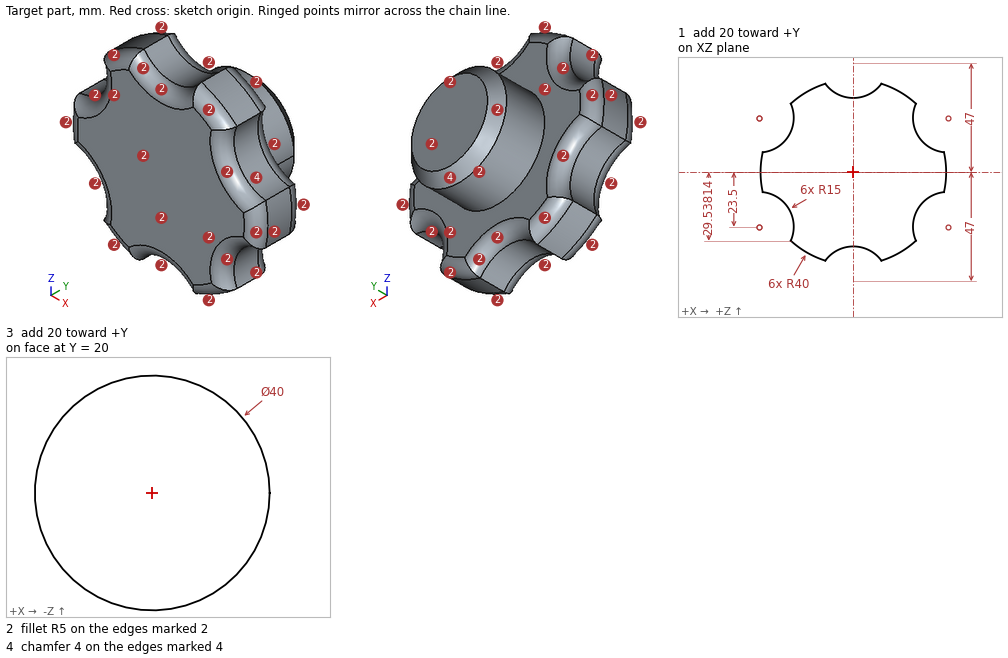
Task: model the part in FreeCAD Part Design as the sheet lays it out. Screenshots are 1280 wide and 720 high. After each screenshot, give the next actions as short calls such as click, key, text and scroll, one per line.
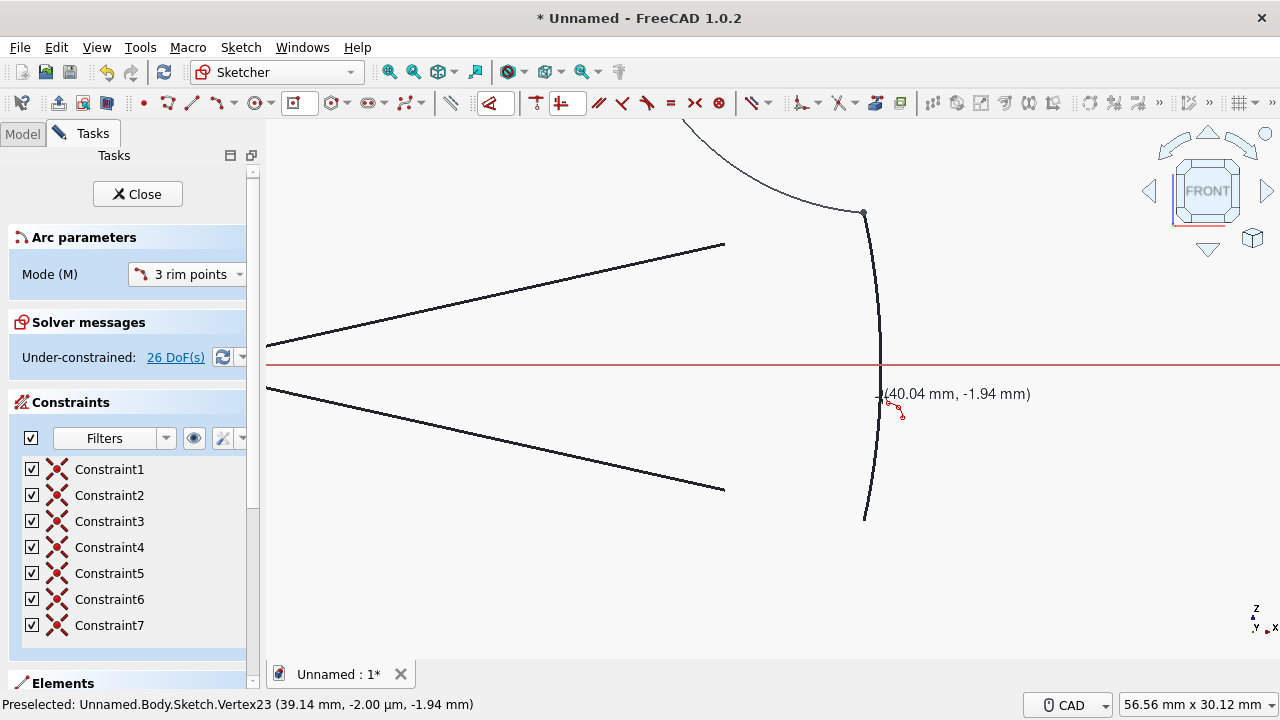
click(879, 396)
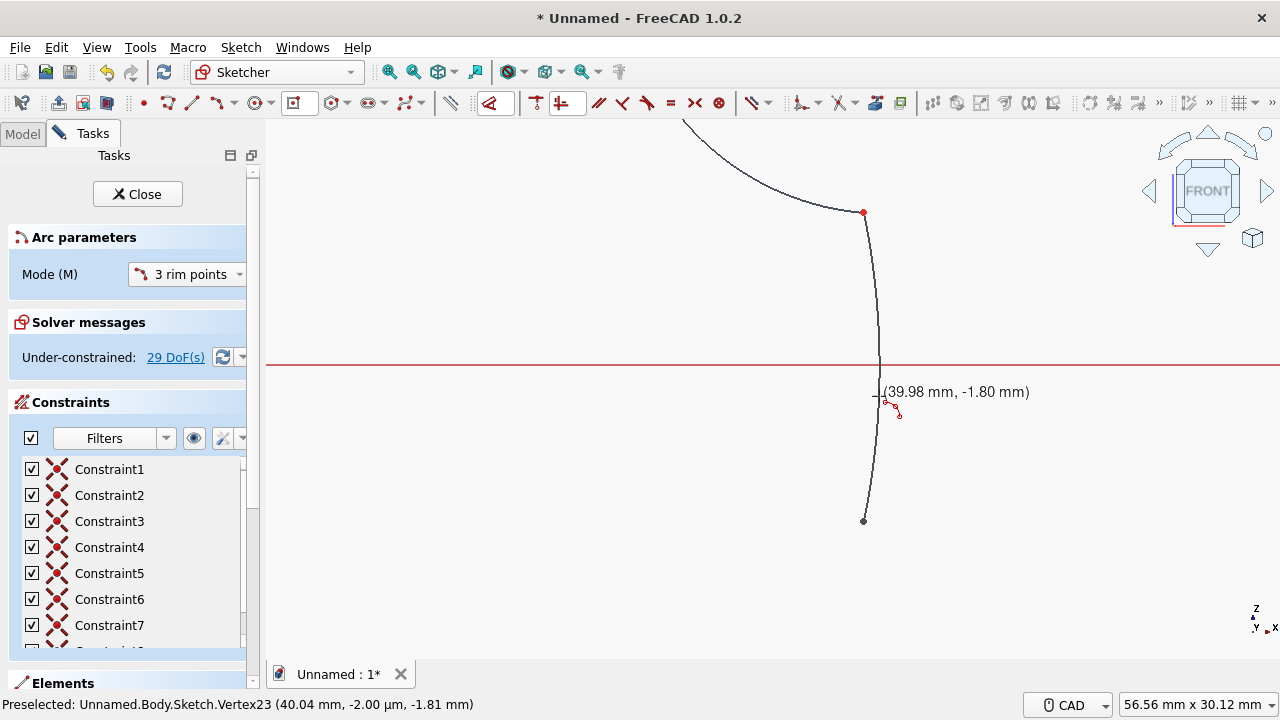
click(864, 521)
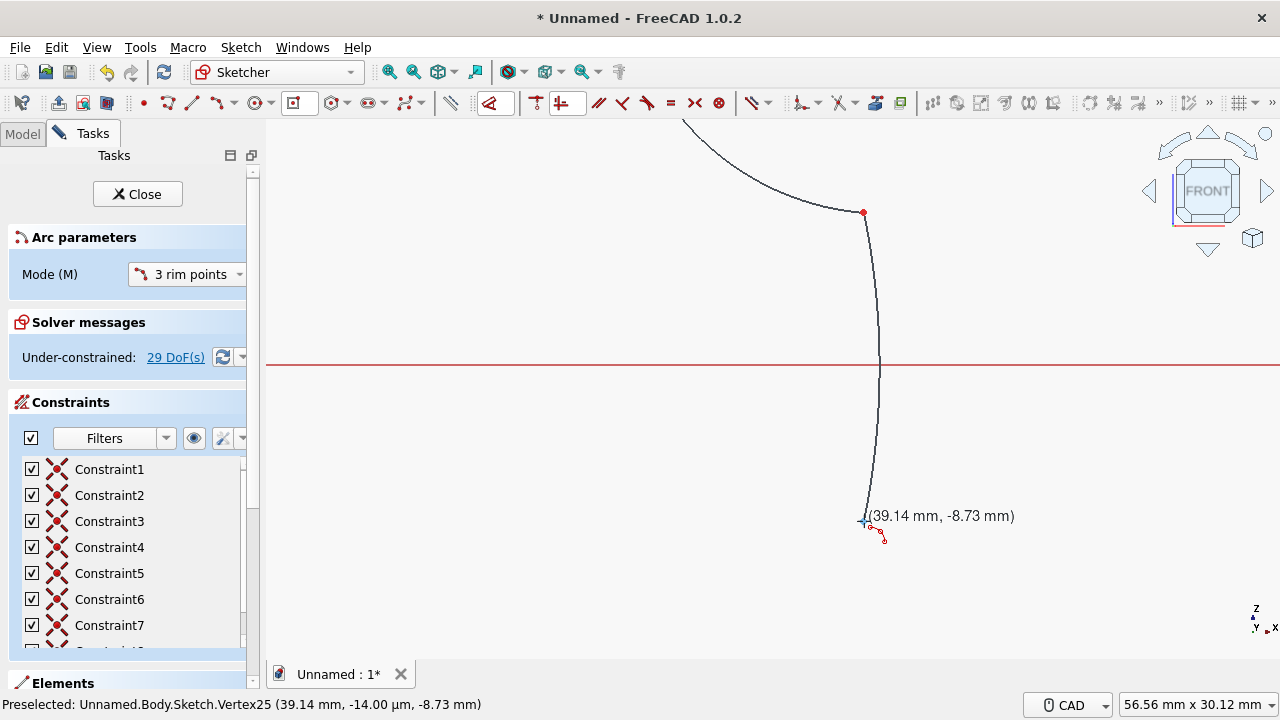
scroll(882, 397, down, 7)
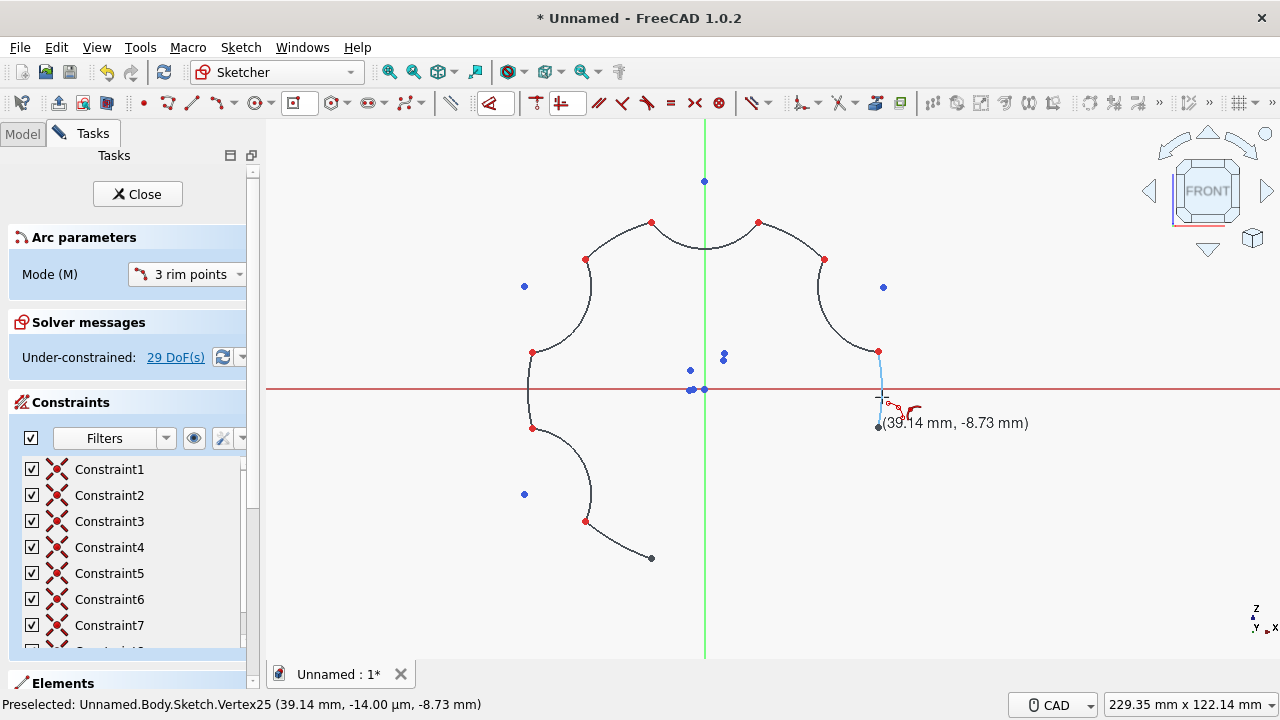
click(824, 520)
click(827, 460)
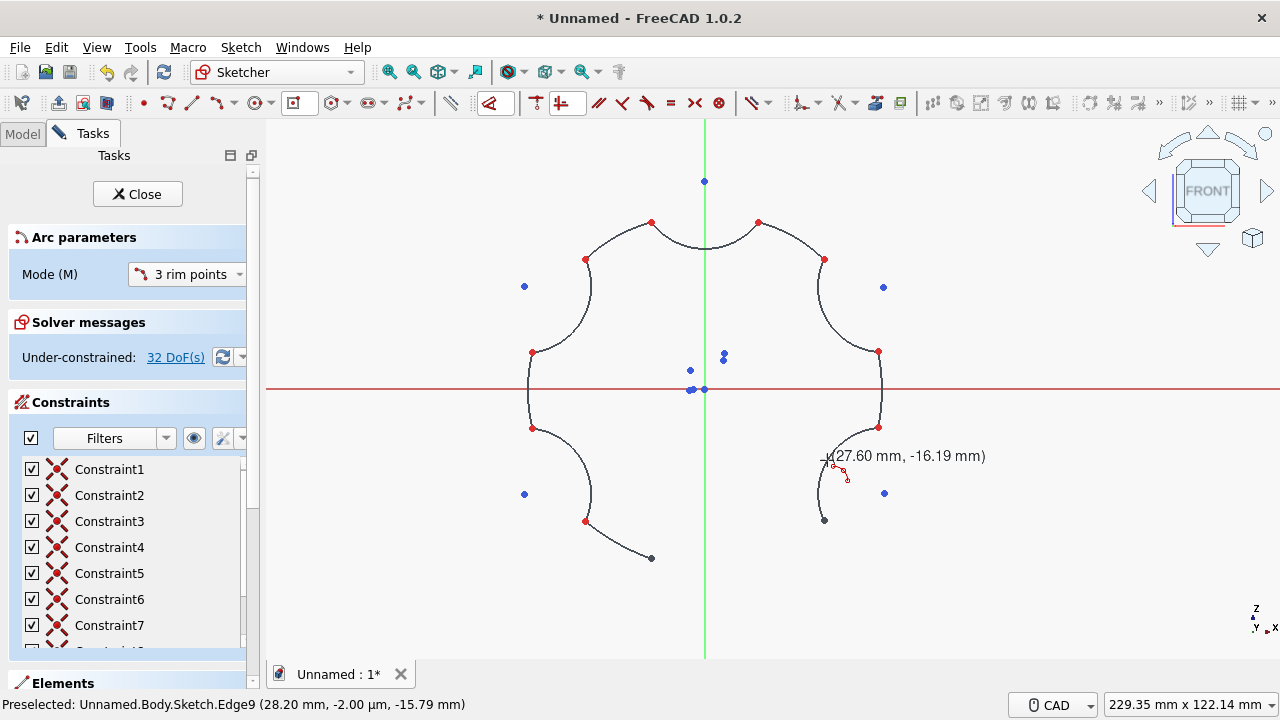
click(824, 521)
click(758, 558)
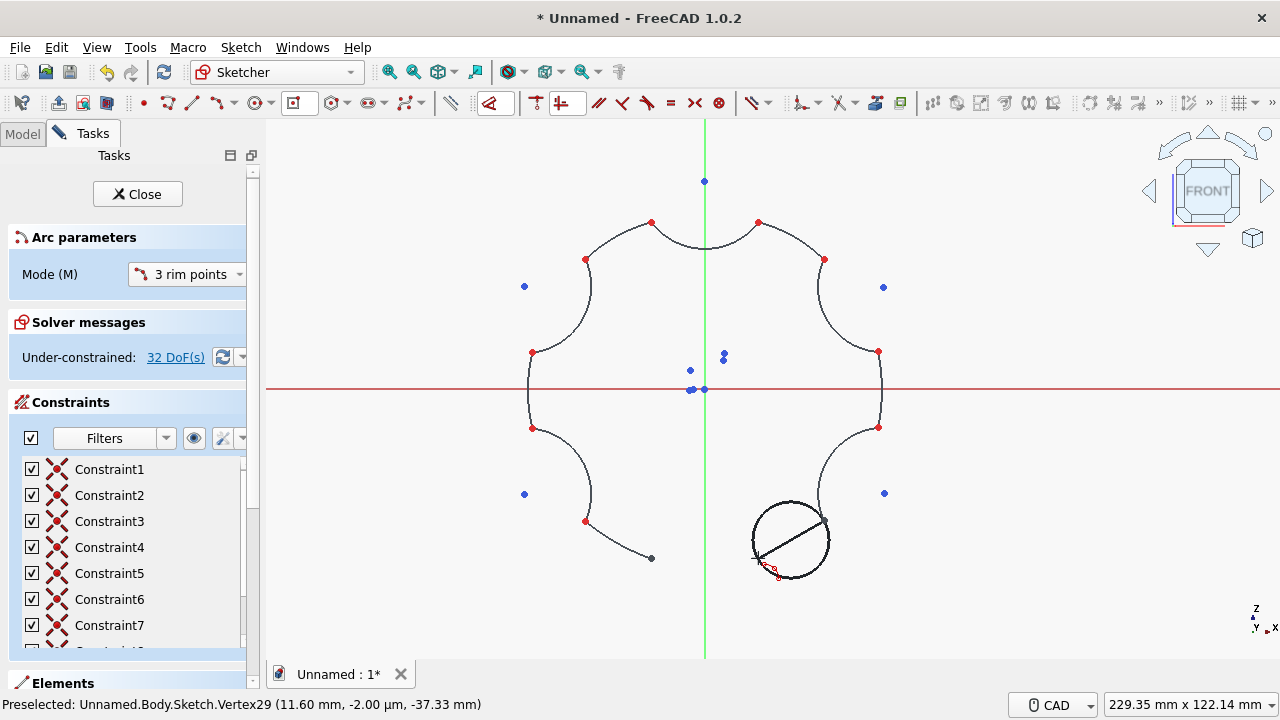
scroll(793, 543, up, 7)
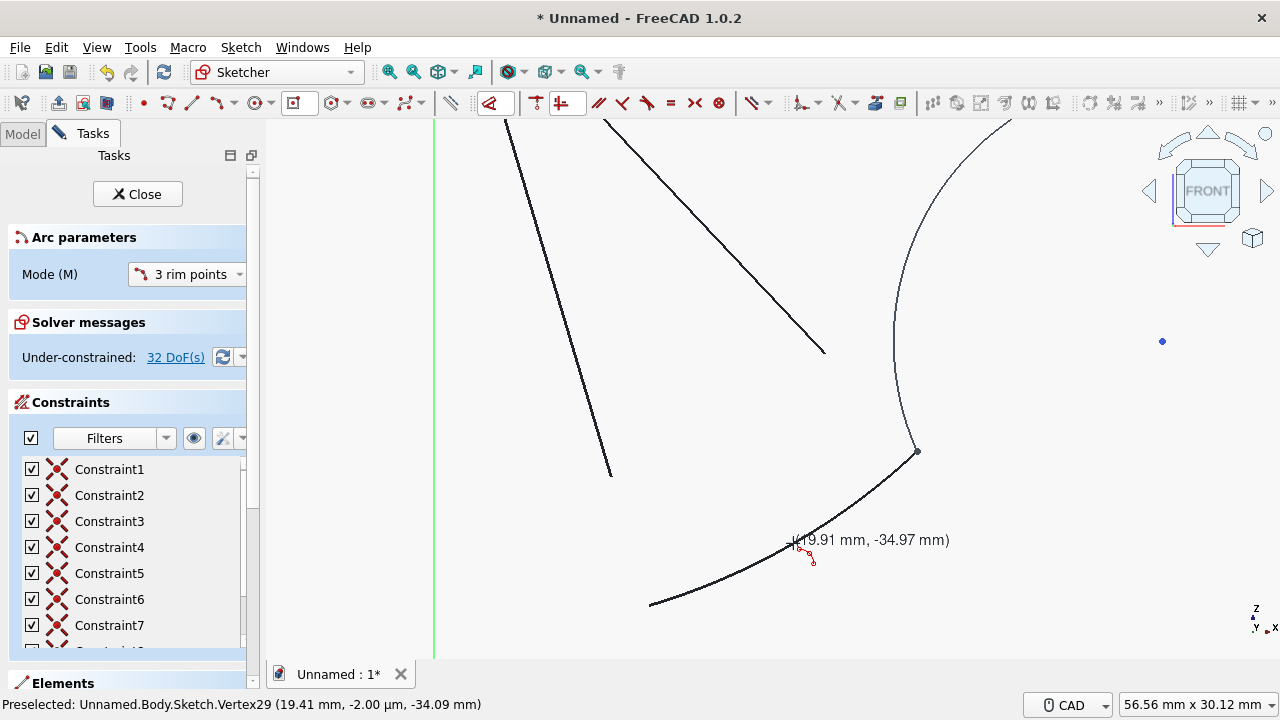
click(793, 539)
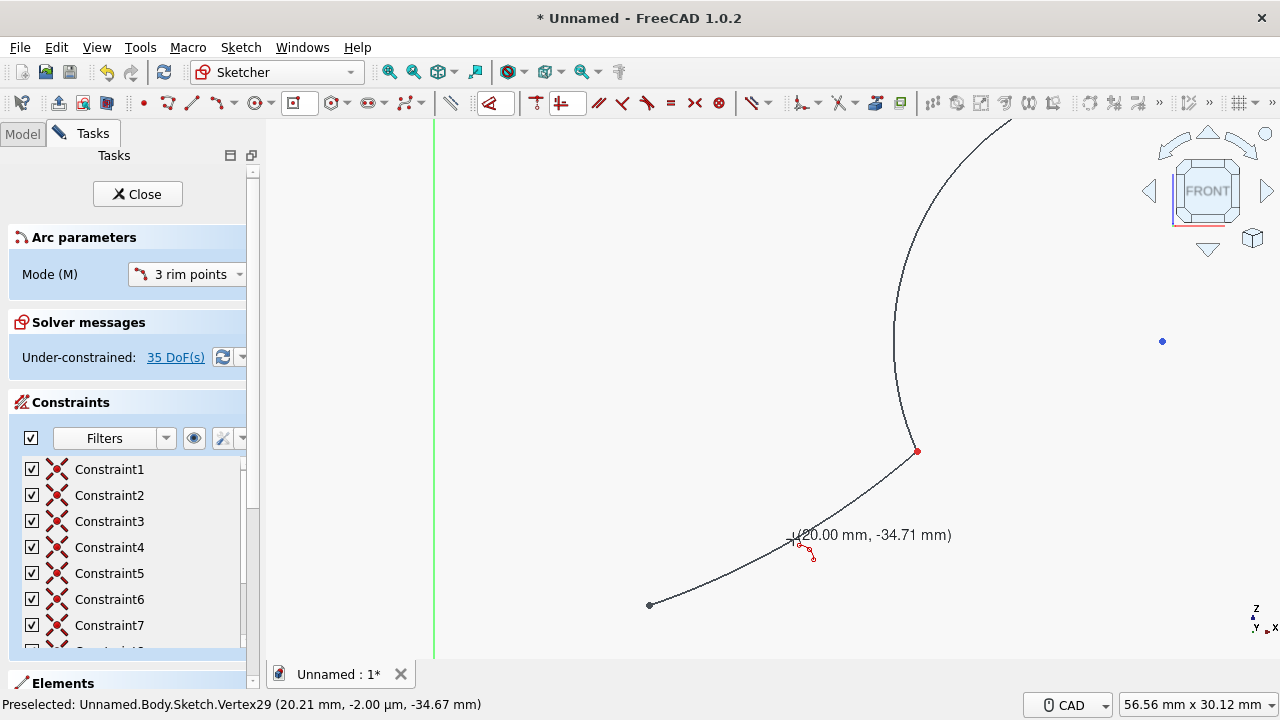
click(649, 605)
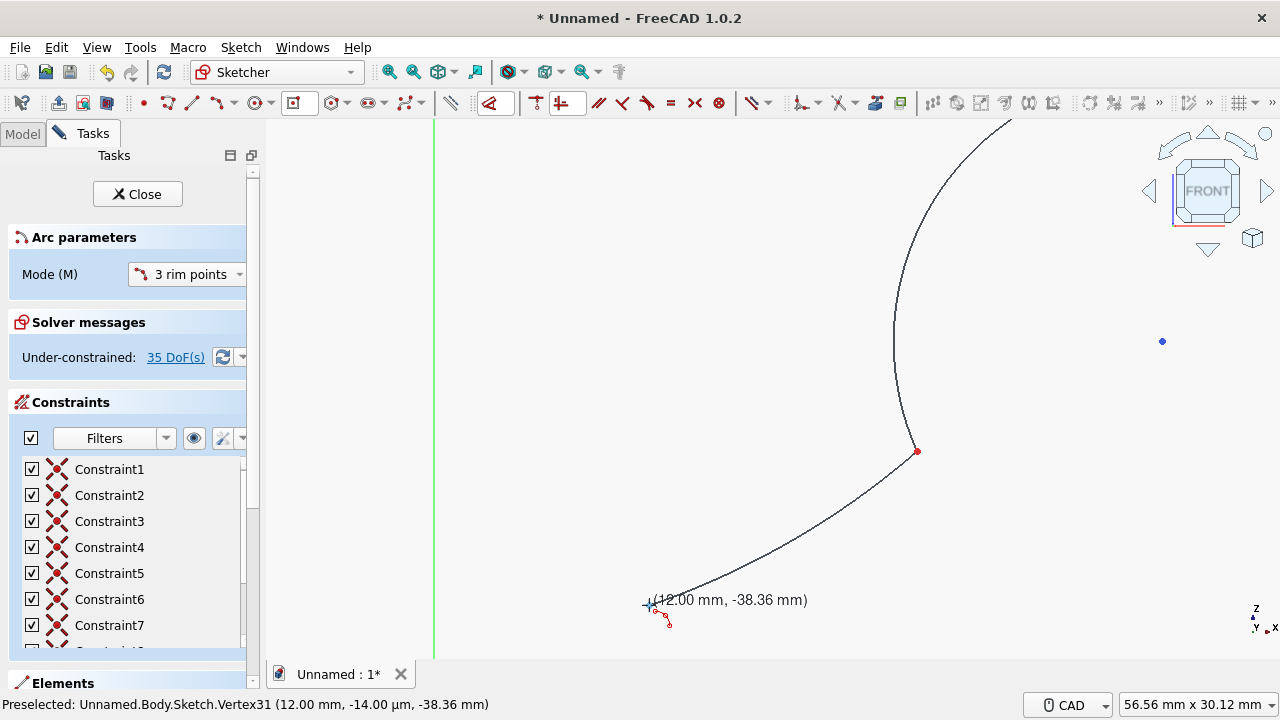
scroll(793, 543, down, 7)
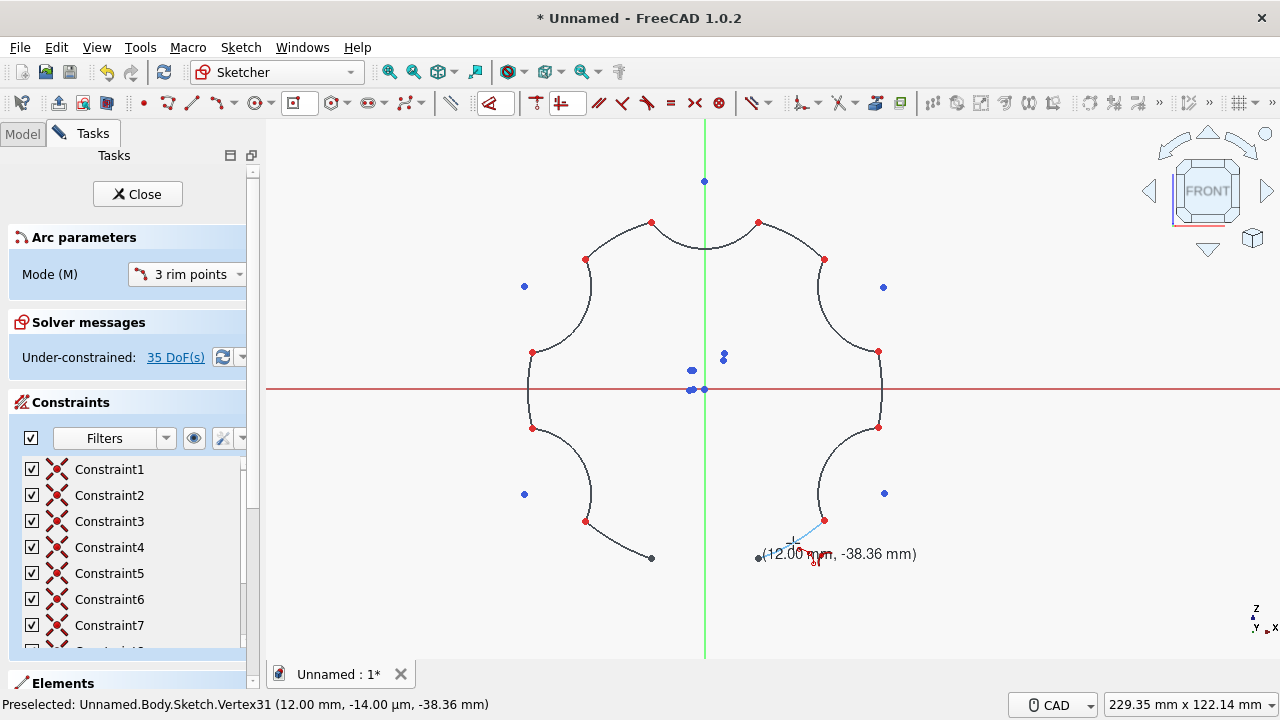
click(652, 559)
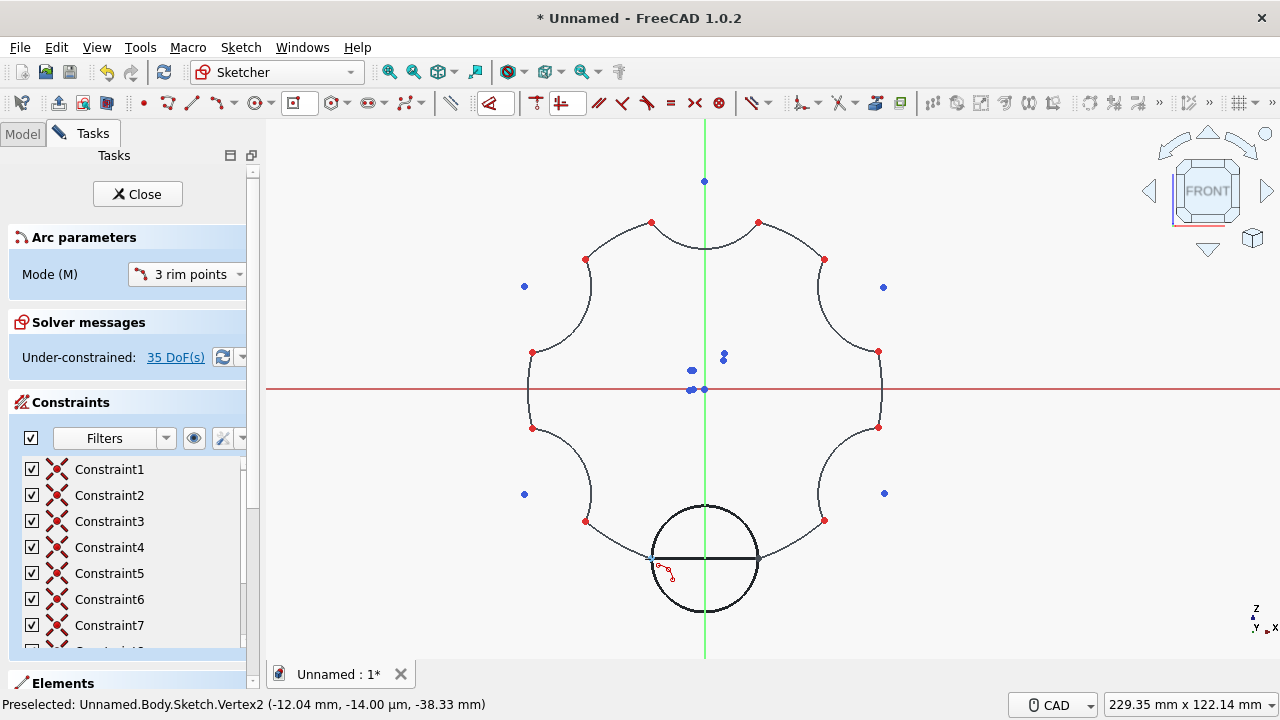
scroll(717, 532, up, 2)